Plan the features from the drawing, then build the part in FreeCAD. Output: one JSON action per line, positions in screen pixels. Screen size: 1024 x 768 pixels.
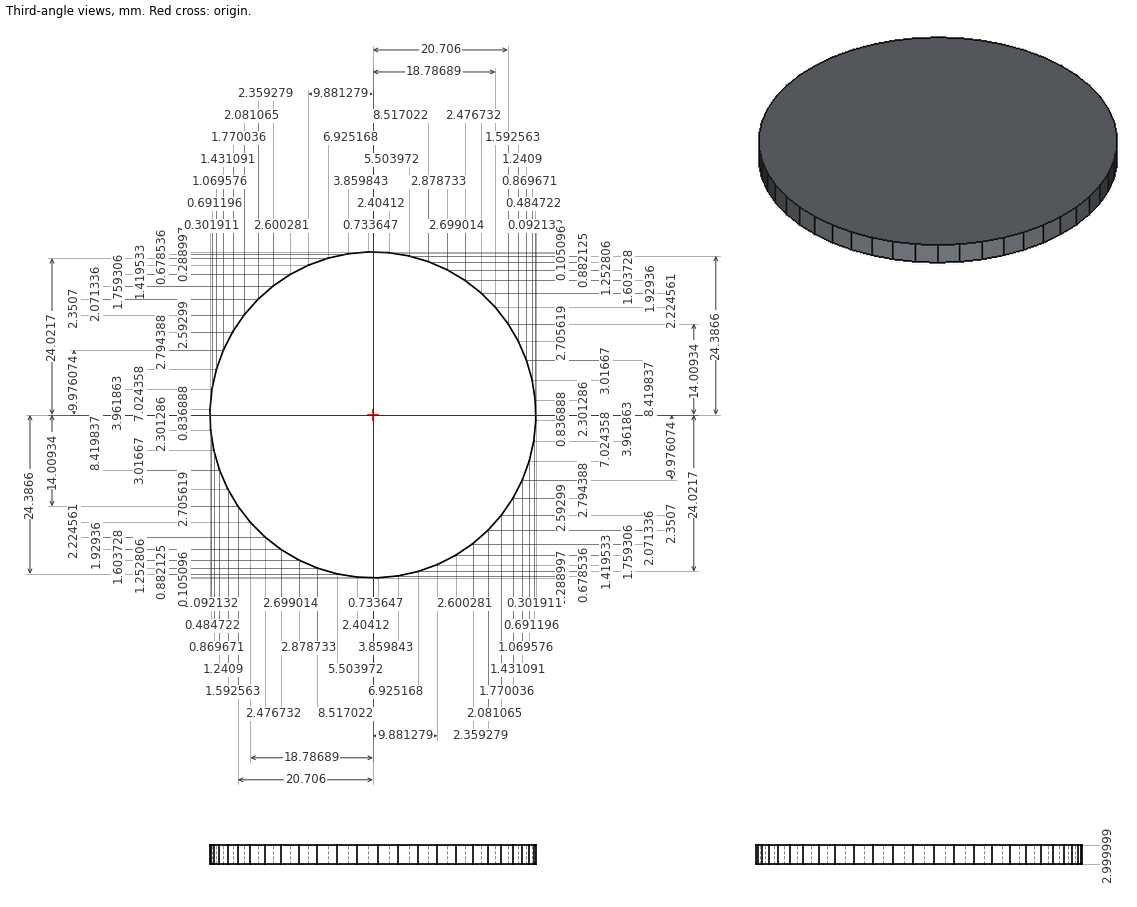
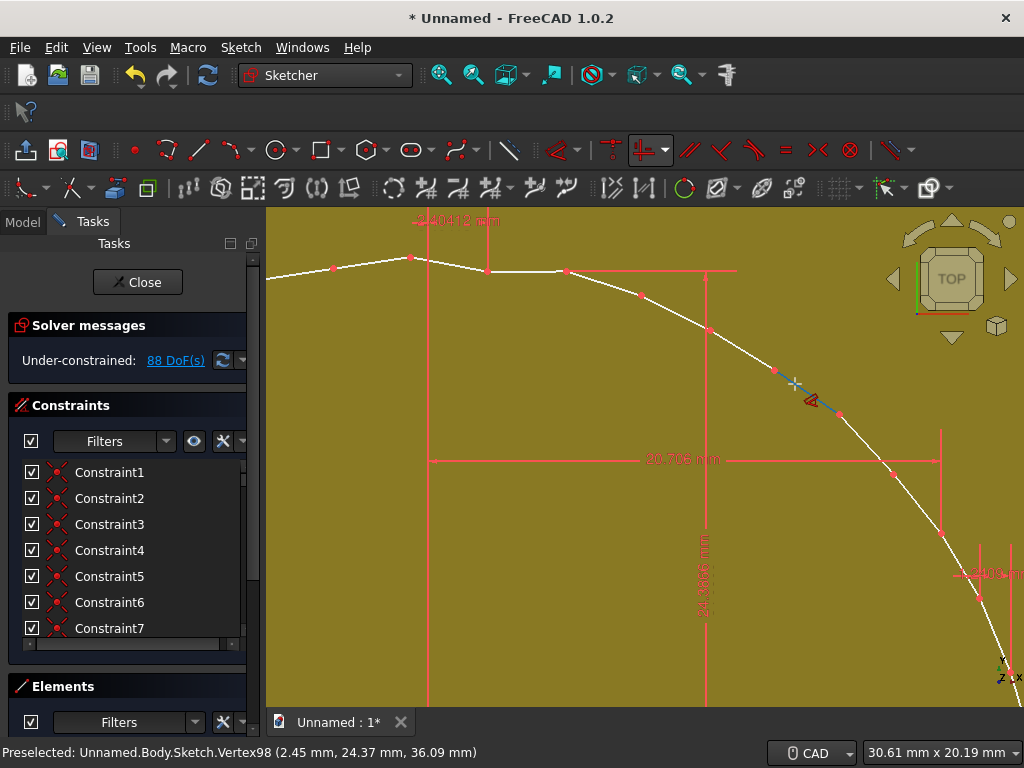
{"action": "left_click", "coordinate": [794, 384]}
{"action": "left_click", "coordinate": [741, 392]}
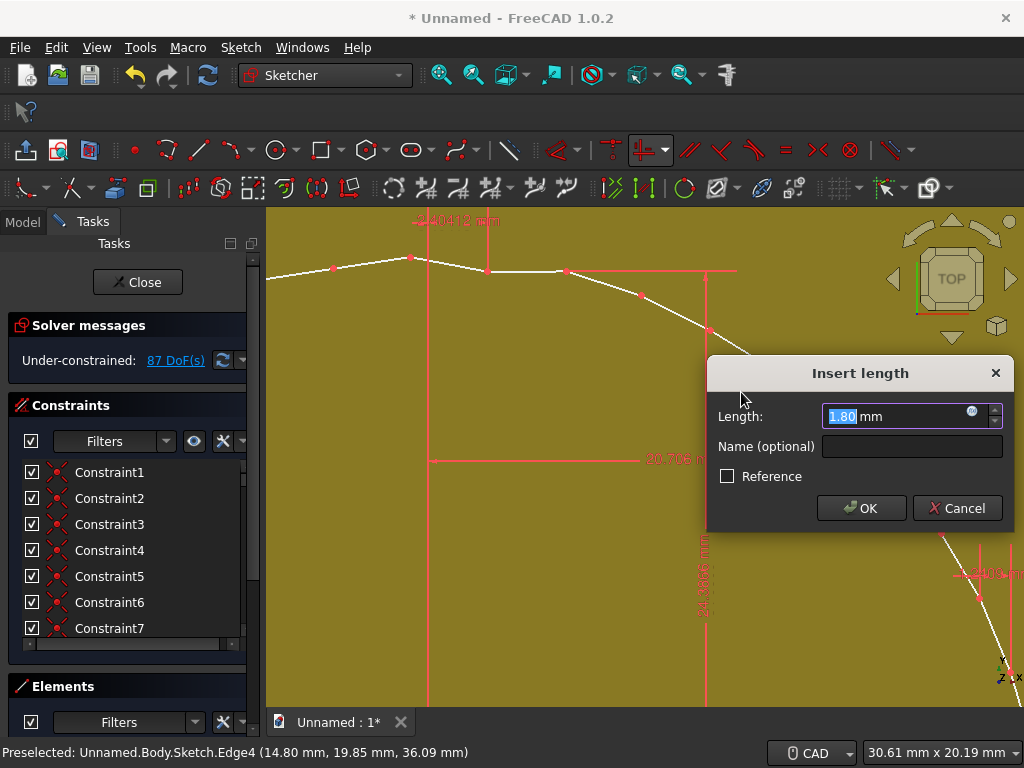
{"action": "type", "text": "1.92936"}
{"action": "key", "text": "Return"}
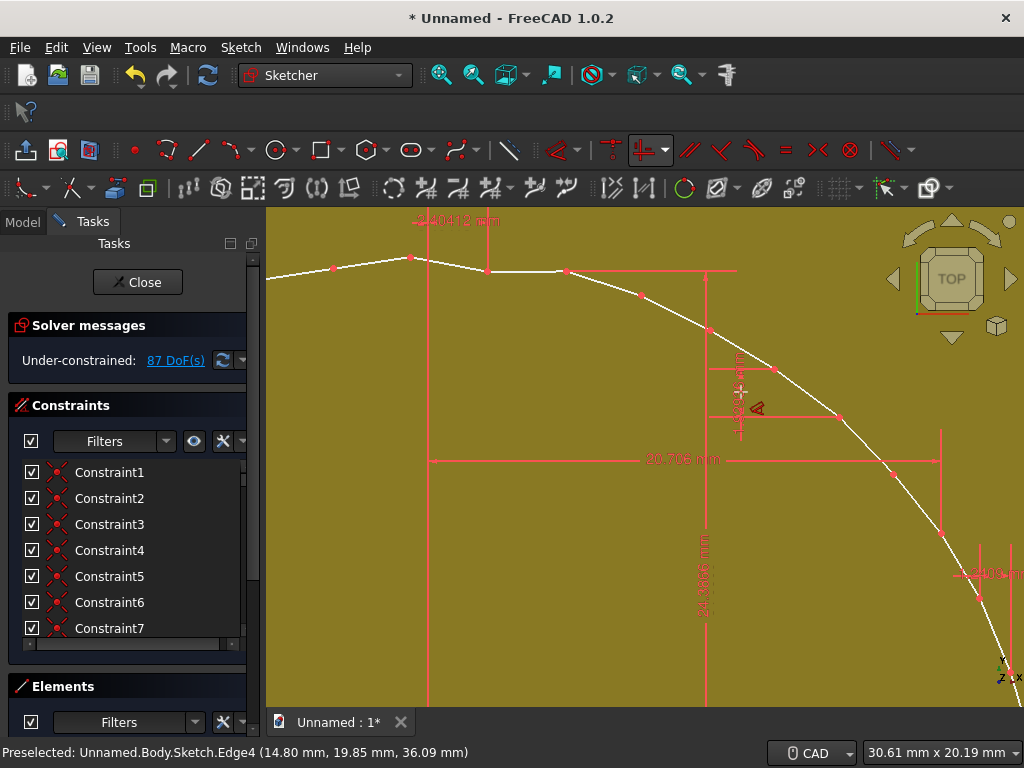
{"action": "scroll", "coordinate": [625, 320], "scroll_direction": "down", "scroll_amount": 7}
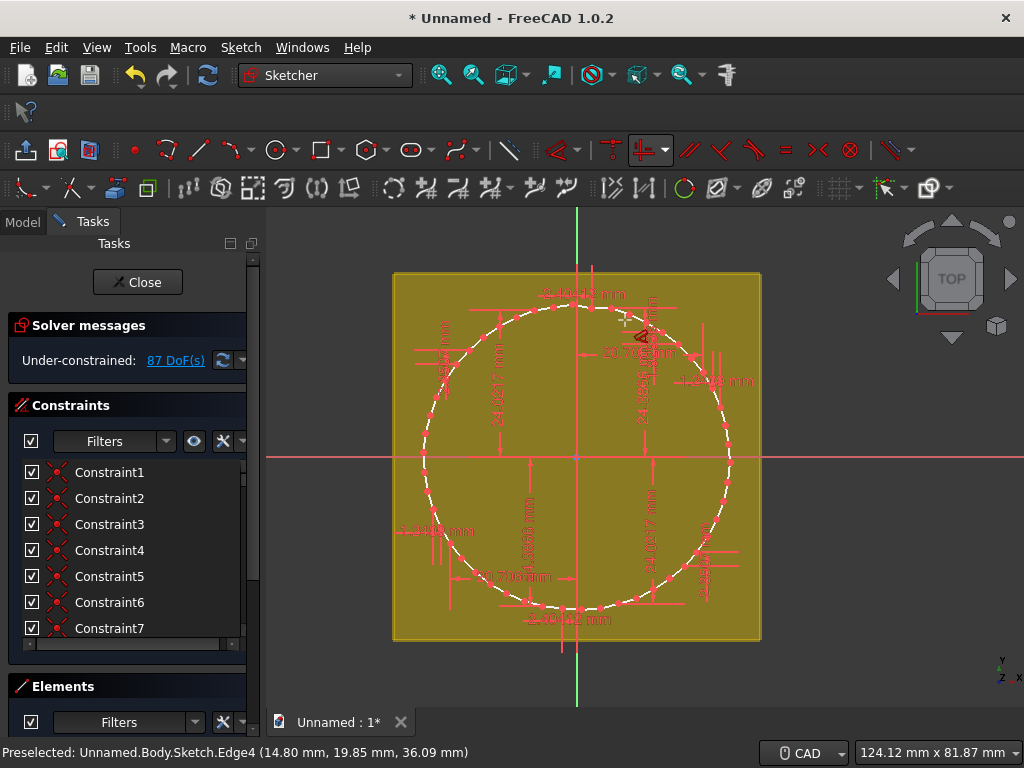
{"action": "scroll", "coordinate": [722, 413], "scroll_direction": "up", "scroll_amount": 5}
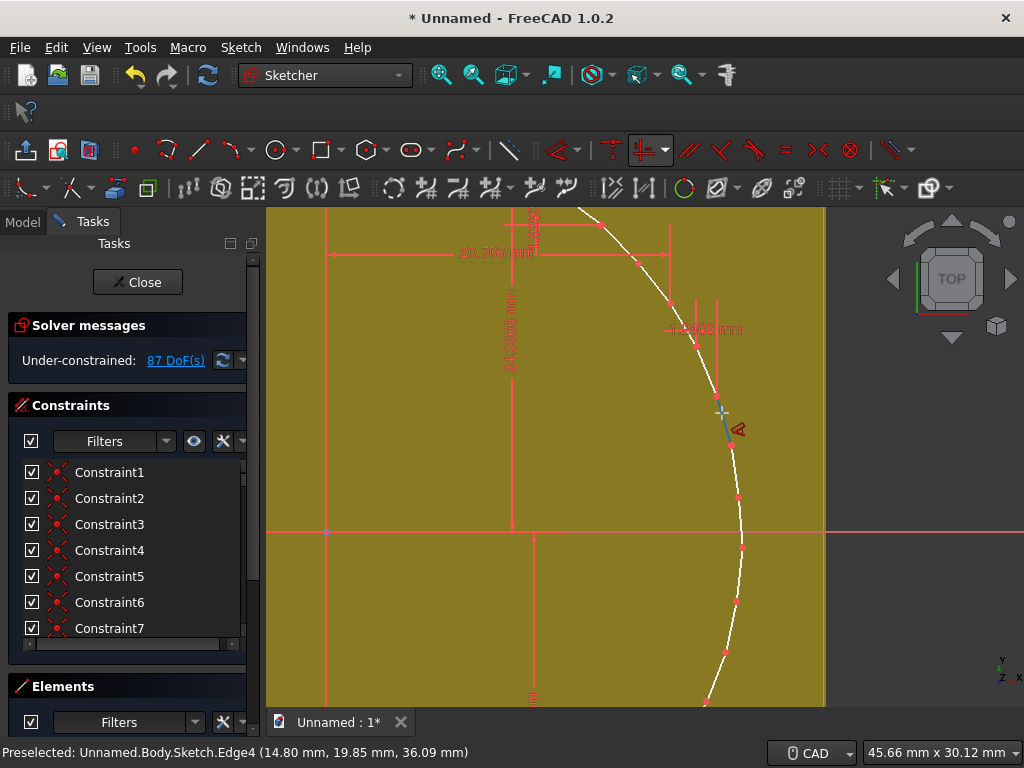
{"action": "left_click", "coordinate": [721, 411]}
{"action": "left_click", "coordinate": [765, 421]}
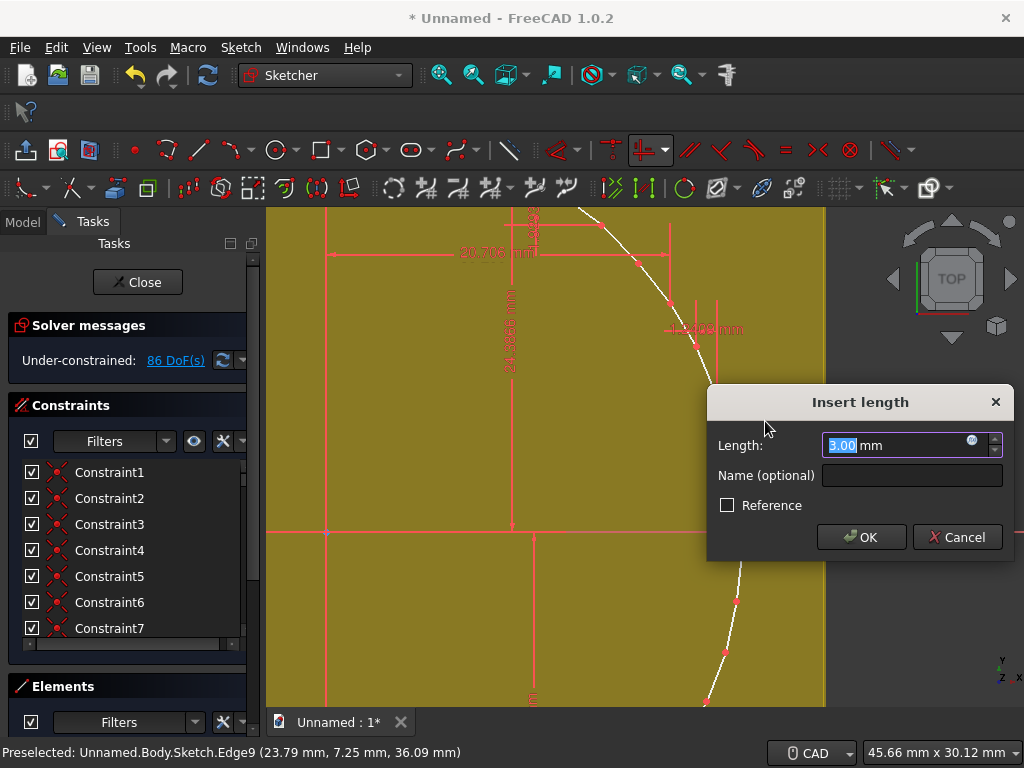
{"action": "type", "text": "3.01667"}
{"action": "key", "text": "Return"}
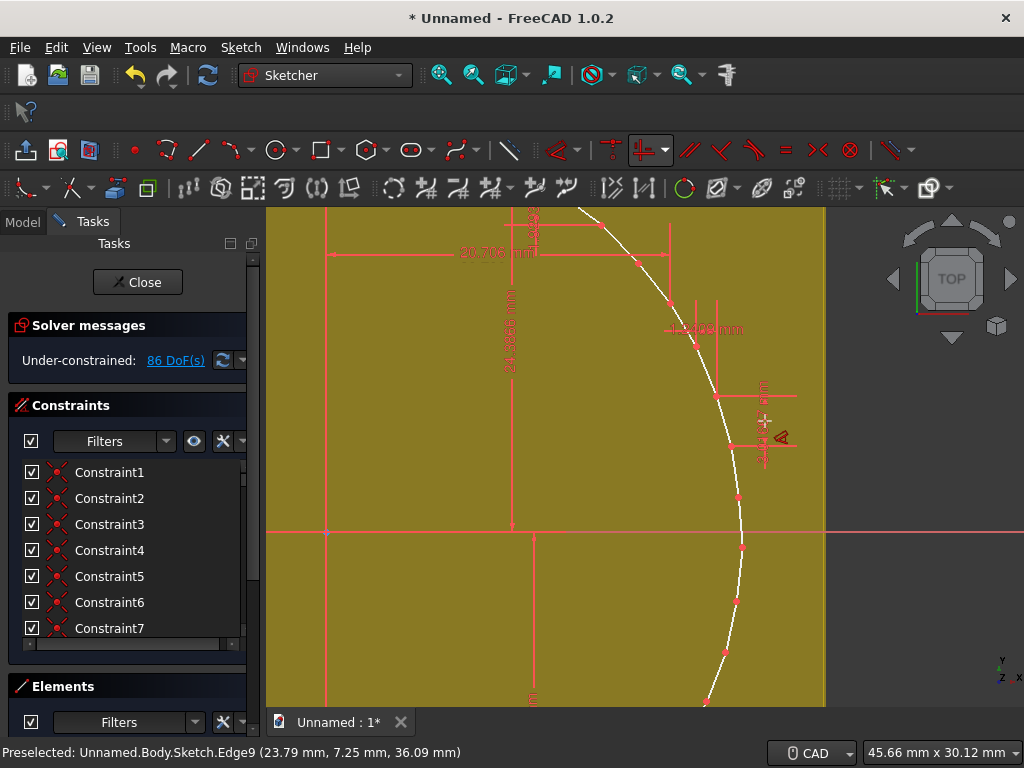
{"action": "scroll", "coordinate": [722, 413], "scroll_direction": "down", "scroll_amount": 5}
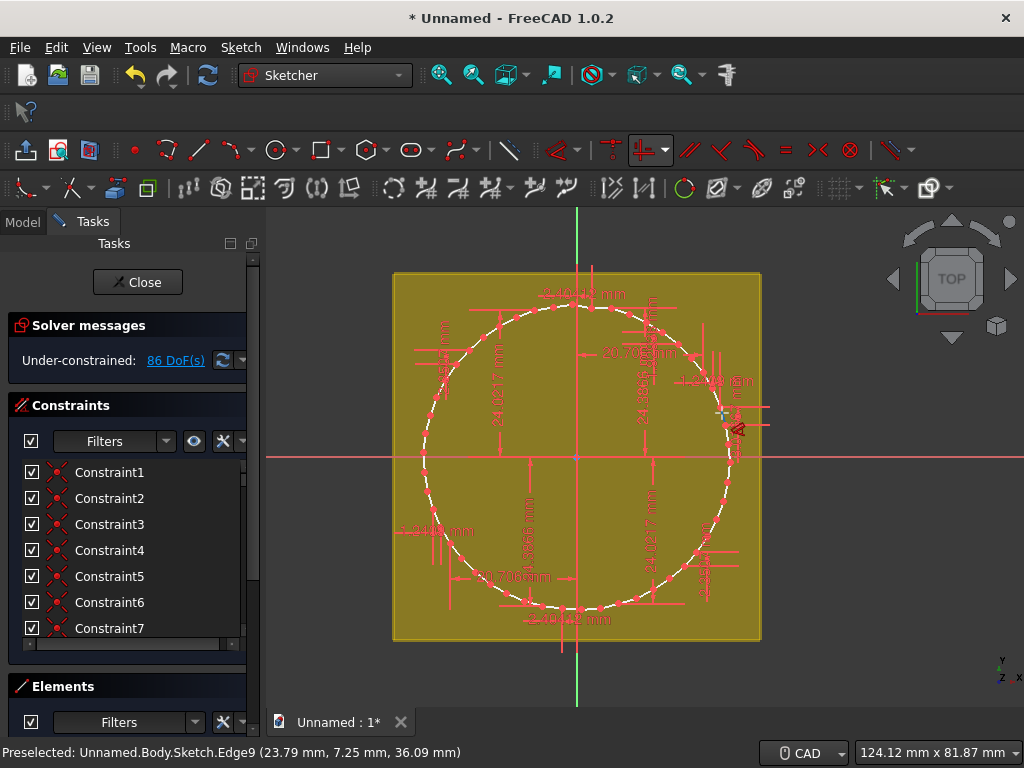
{"action": "scroll", "coordinate": [705, 541], "scroll_direction": "up", "scroll_amount": 5}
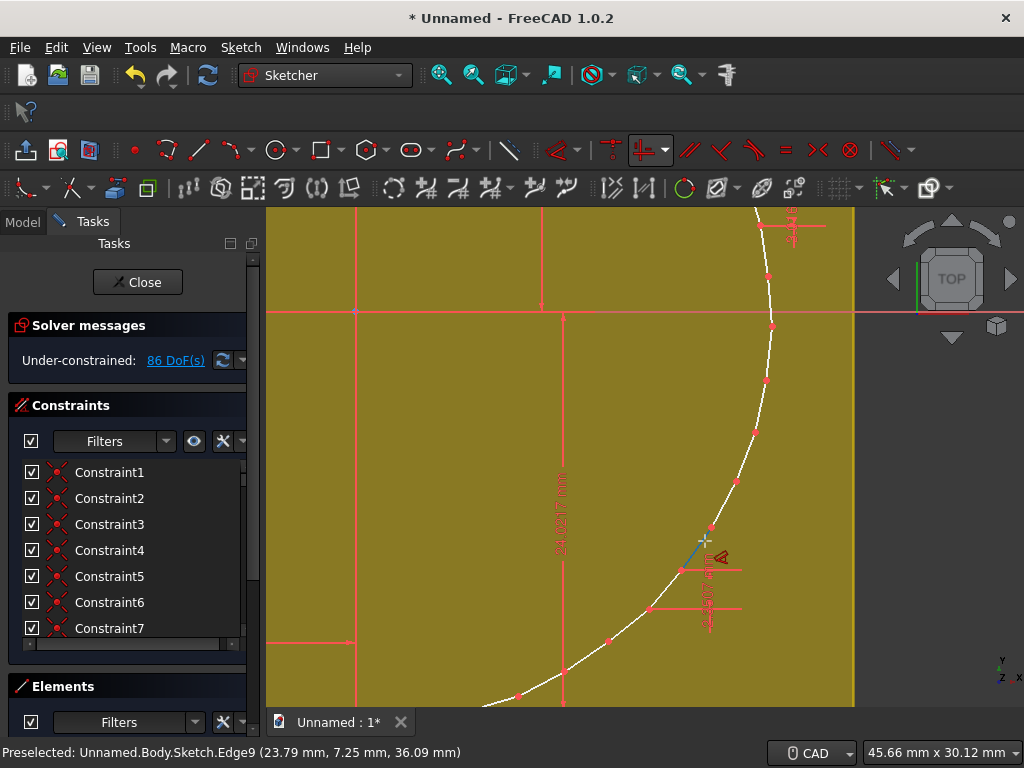
{"action": "left_click", "coordinate": [703, 540]}
{"action": "left_click", "coordinate": [746, 549]}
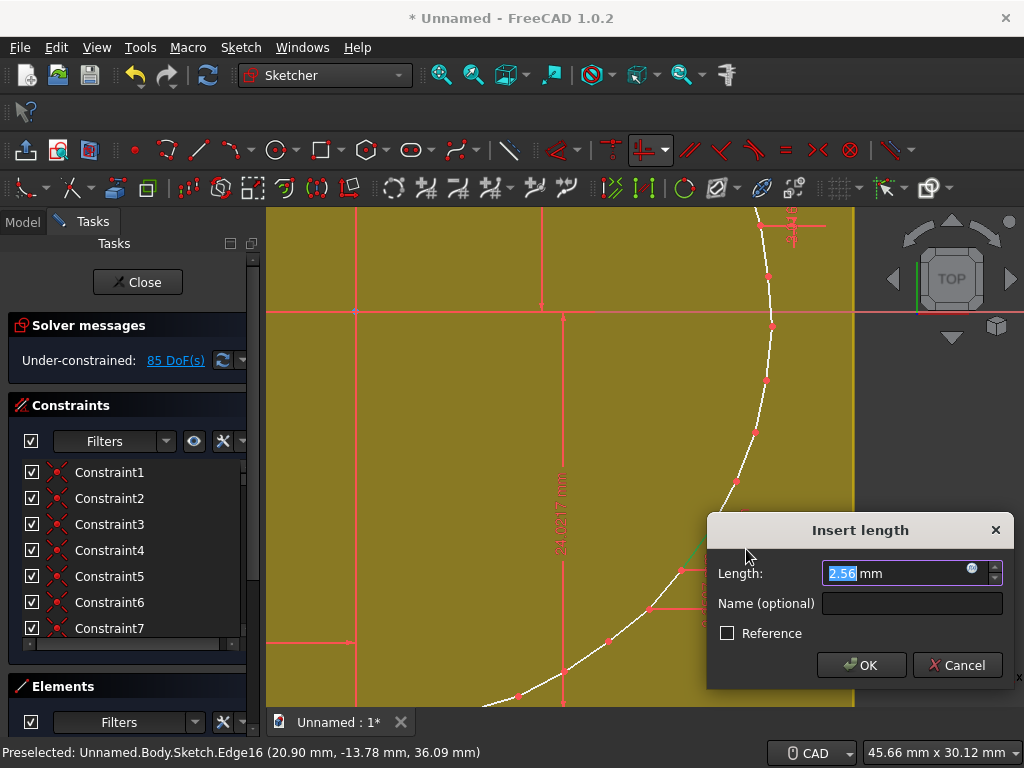
{"action": "type", "text": "2.59299"}
{"action": "key", "text": "Return"}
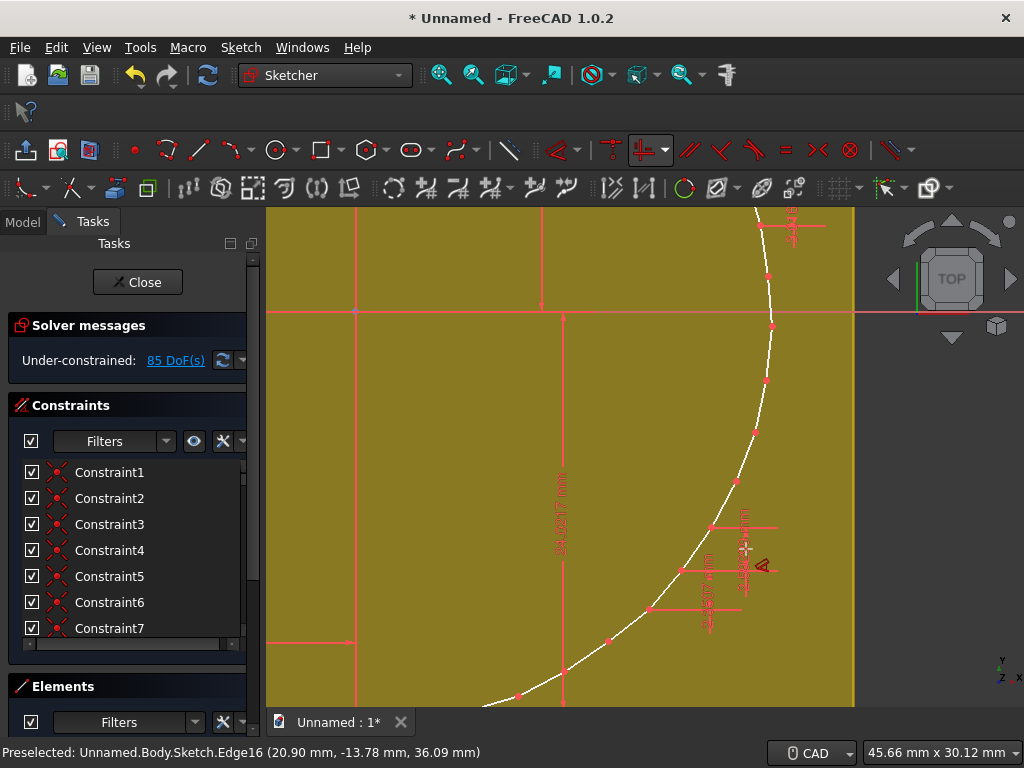
{"action": "scroll", "coordinate": [705, 541], "scroll_direction": "down", "scroll_amount": 5}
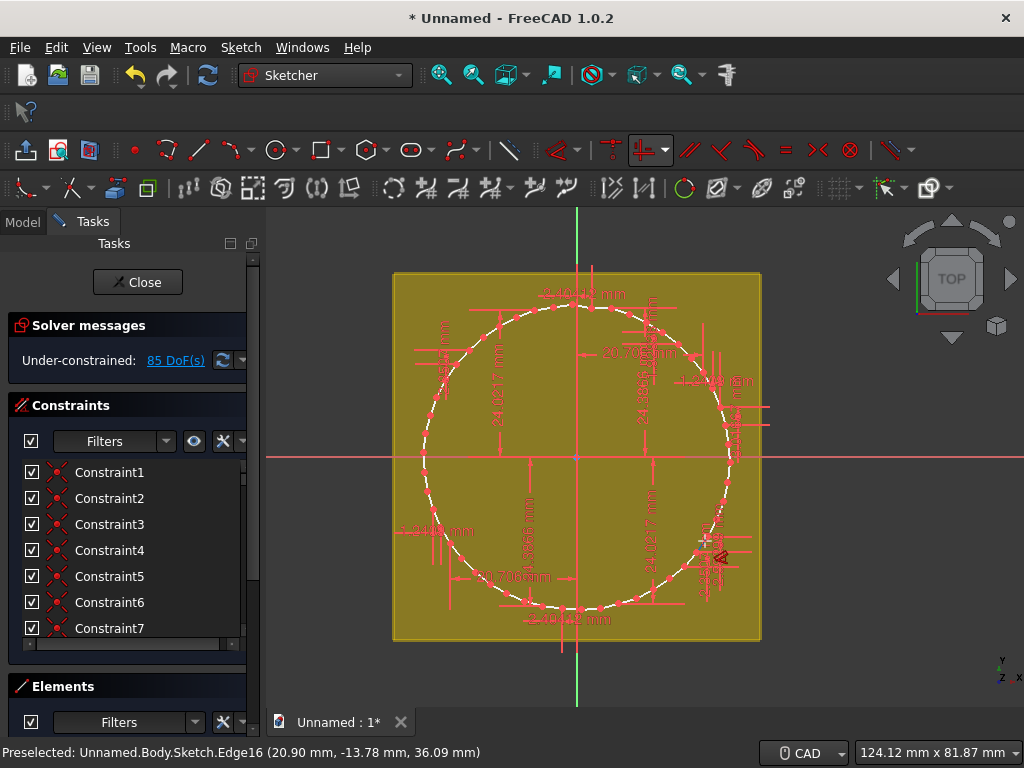
{"action": "scroll", "coordinate": [486, 581], "scroll_direction": "up", "scroll_amount": 7}